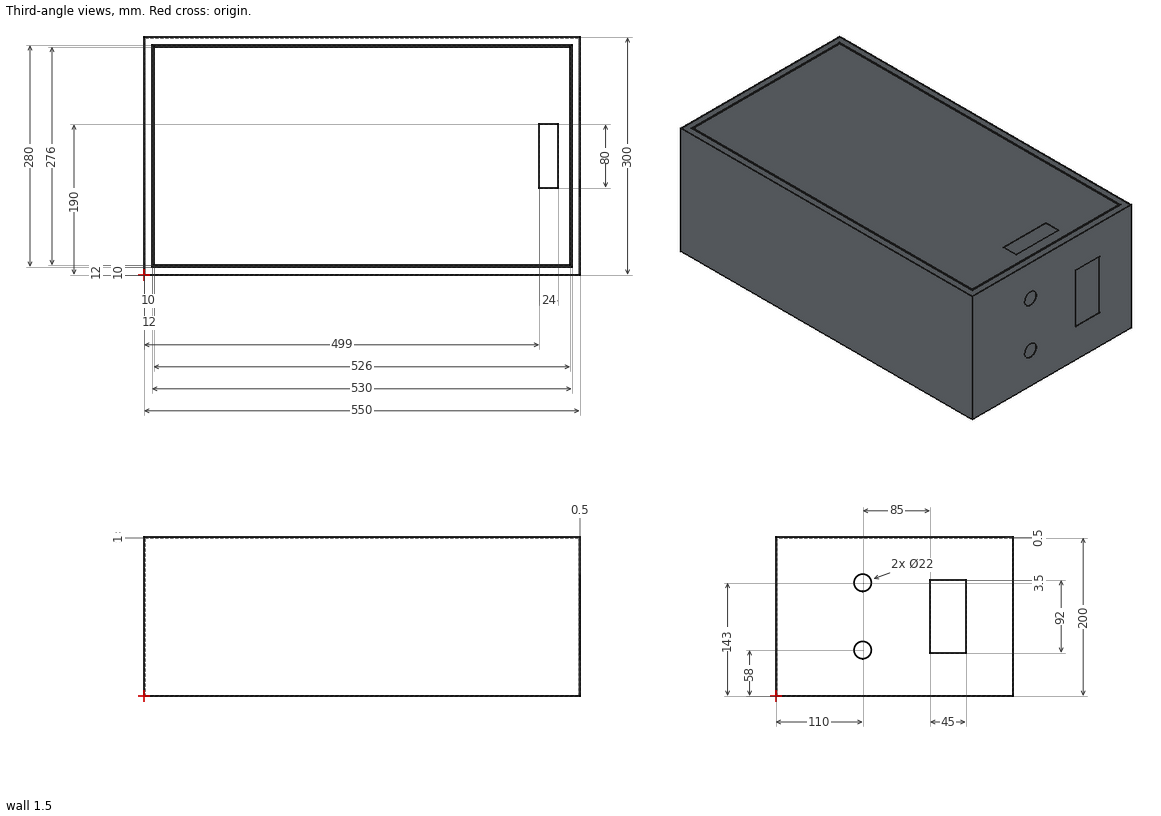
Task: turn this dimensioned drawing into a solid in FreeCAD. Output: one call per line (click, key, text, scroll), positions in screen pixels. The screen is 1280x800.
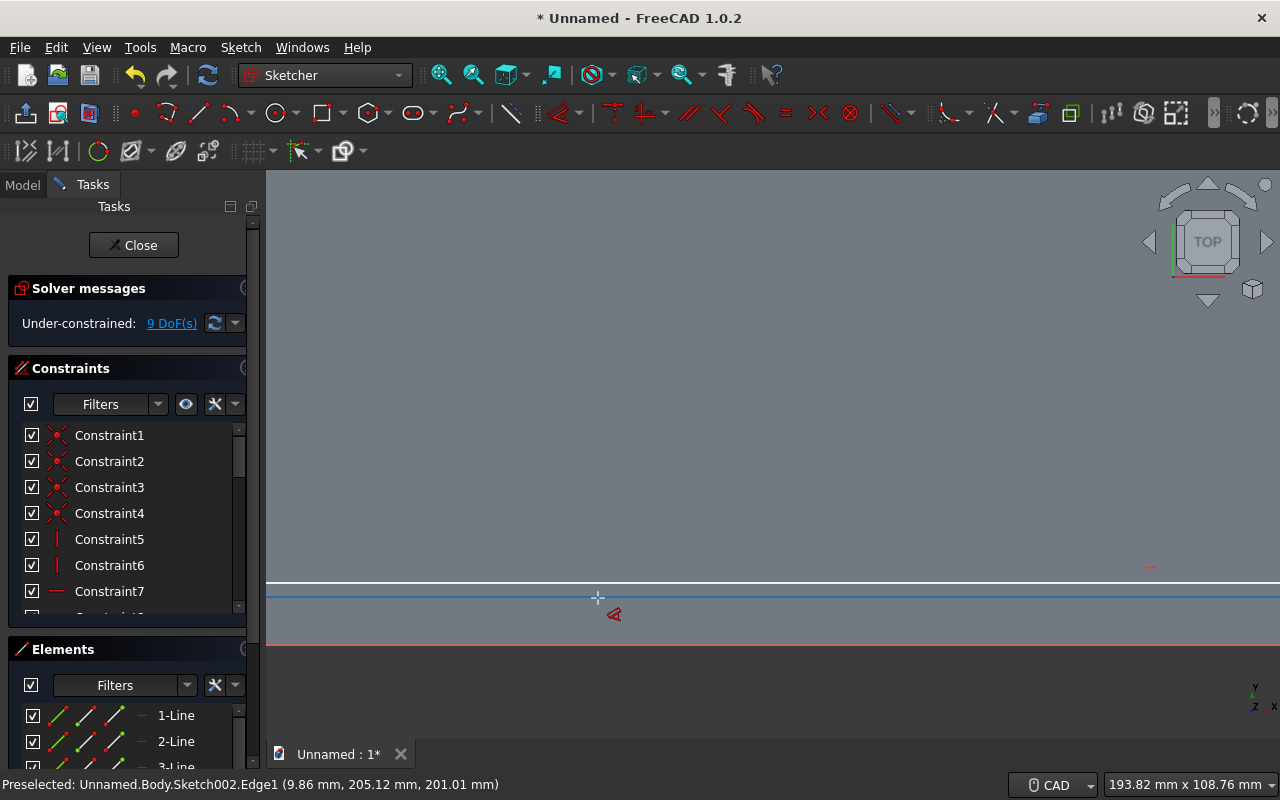
click(598, 597)
click(704, 631)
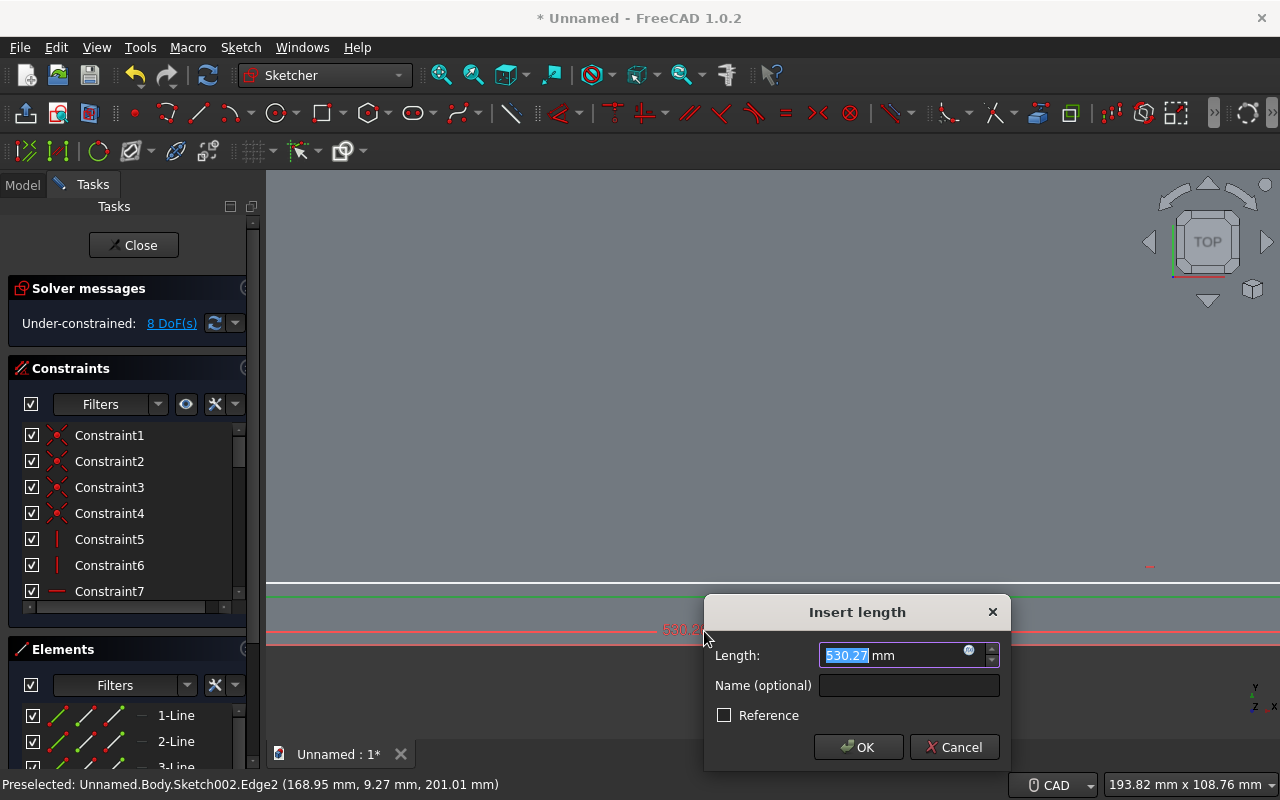
text(530)
key(Return)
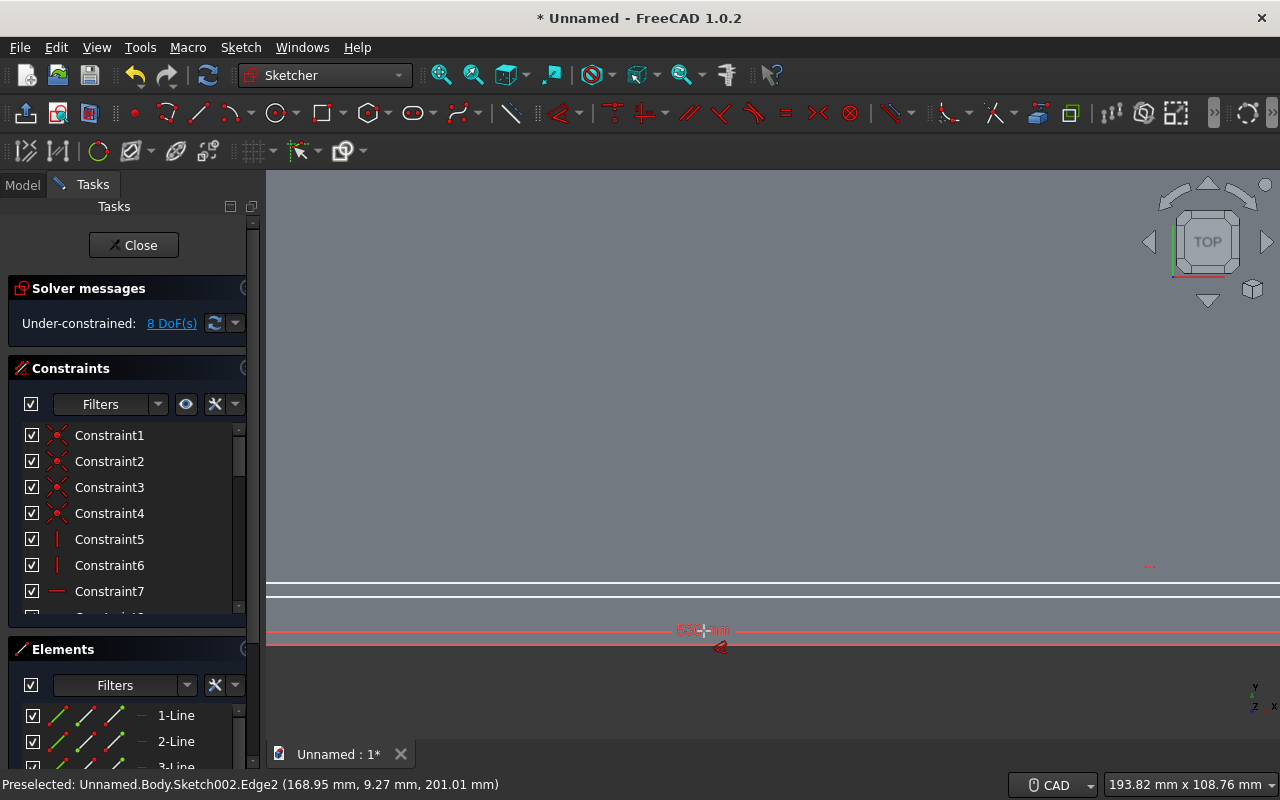
scroll(598, 598, down, 8)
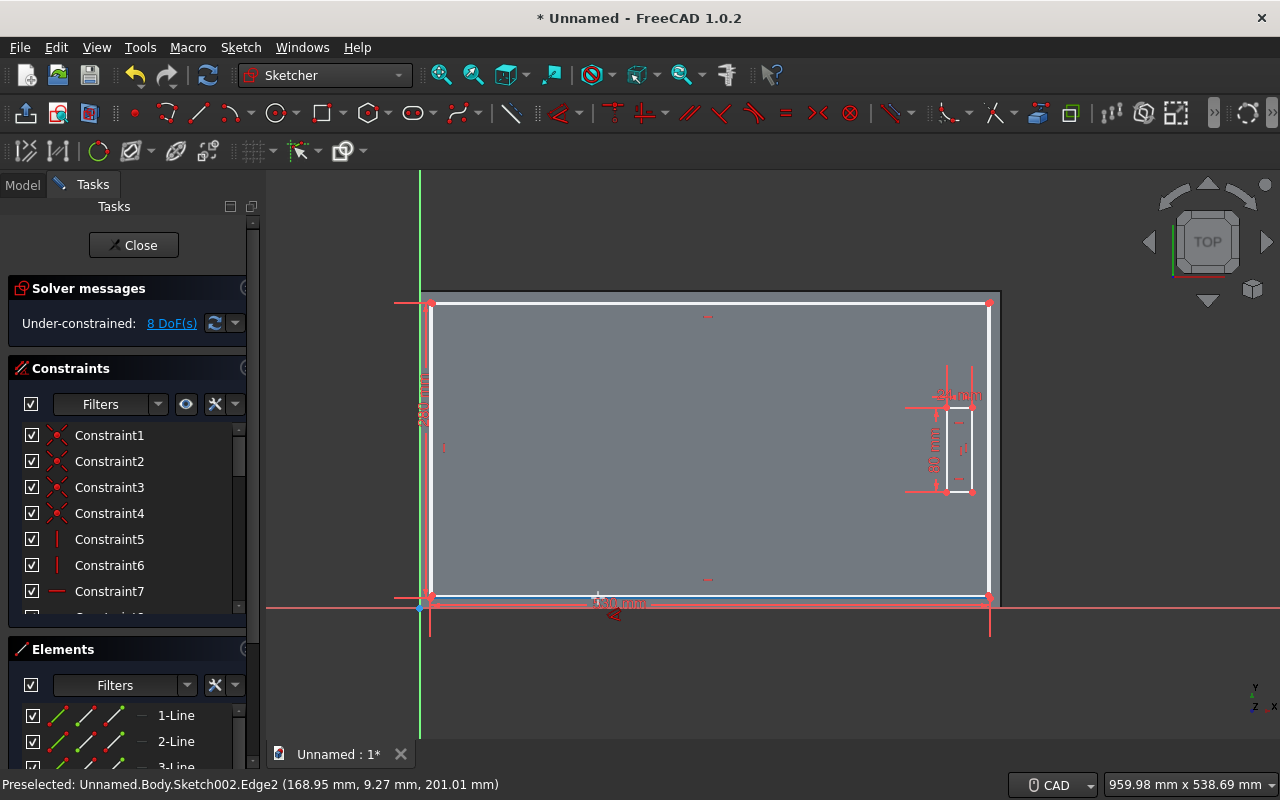
scroll(432, 391, up, 10)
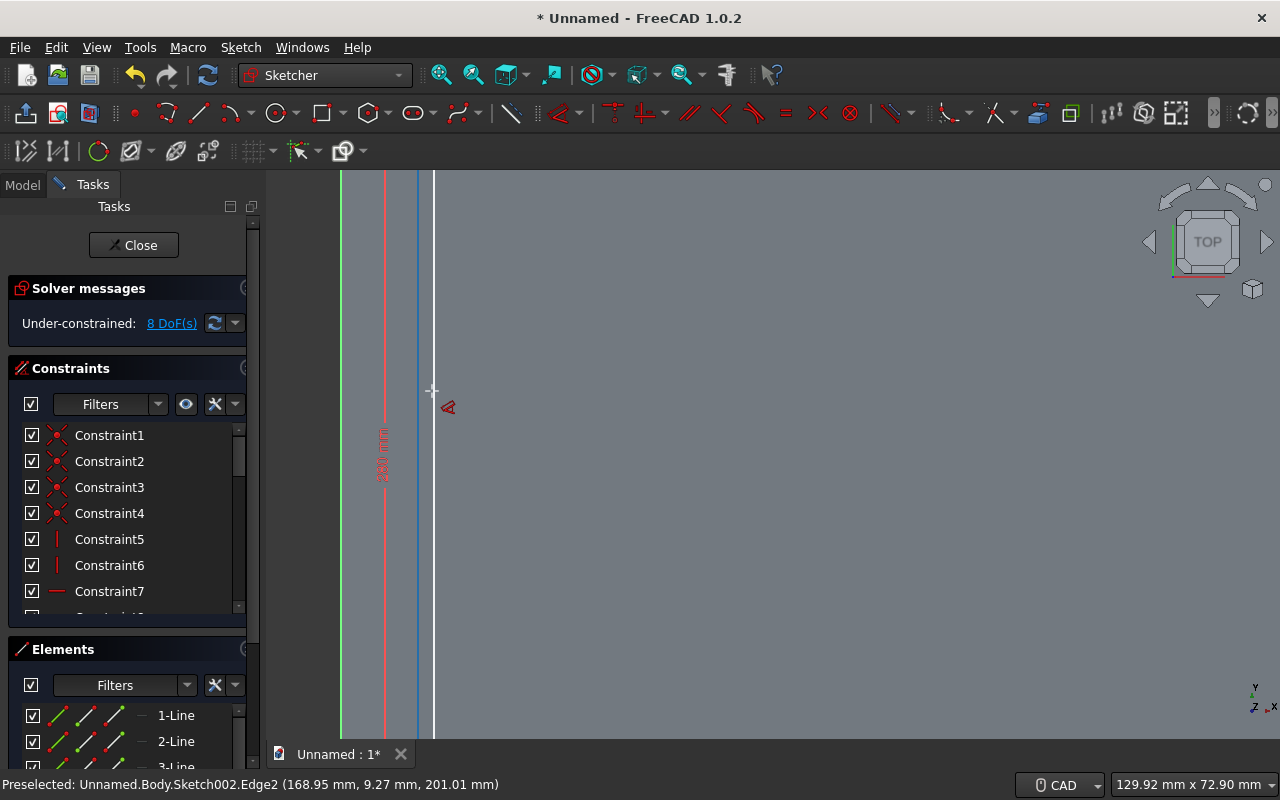
click(434, 392)
click(400, 337)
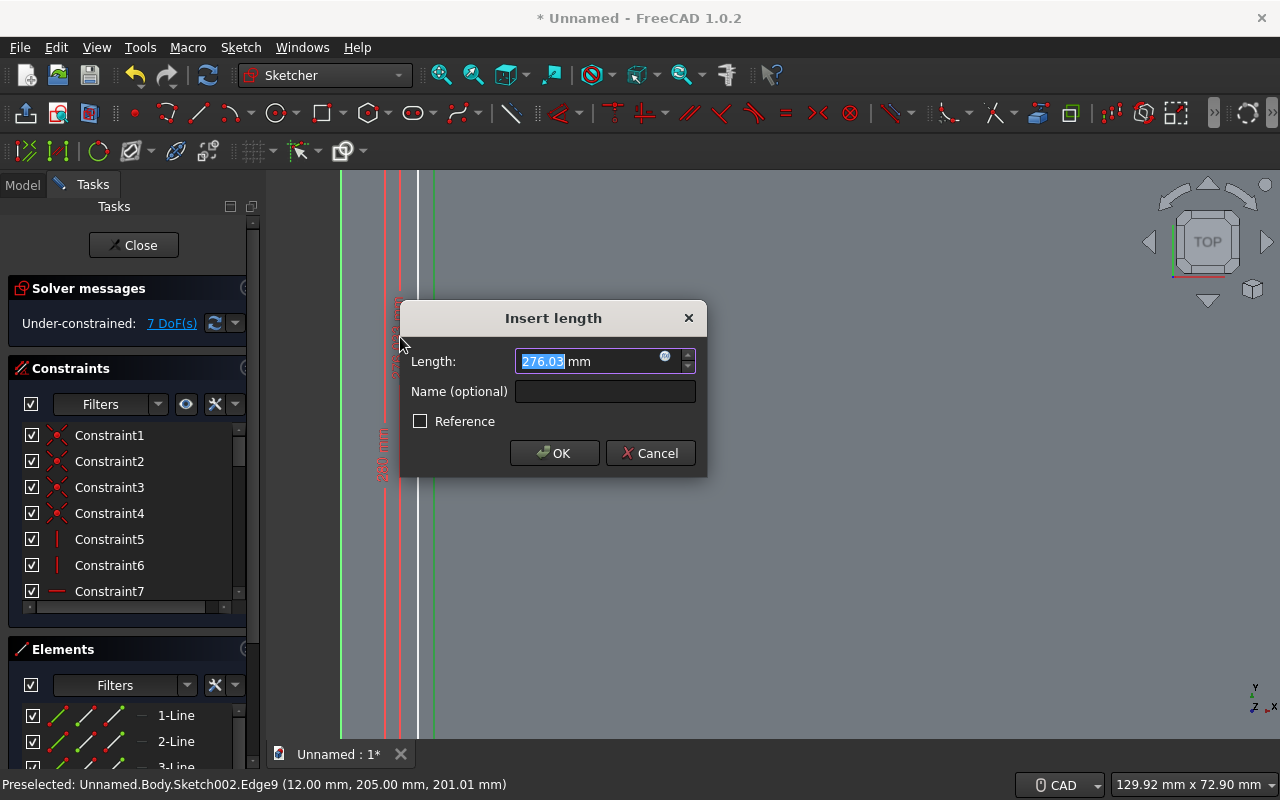
text(276)
key(Return)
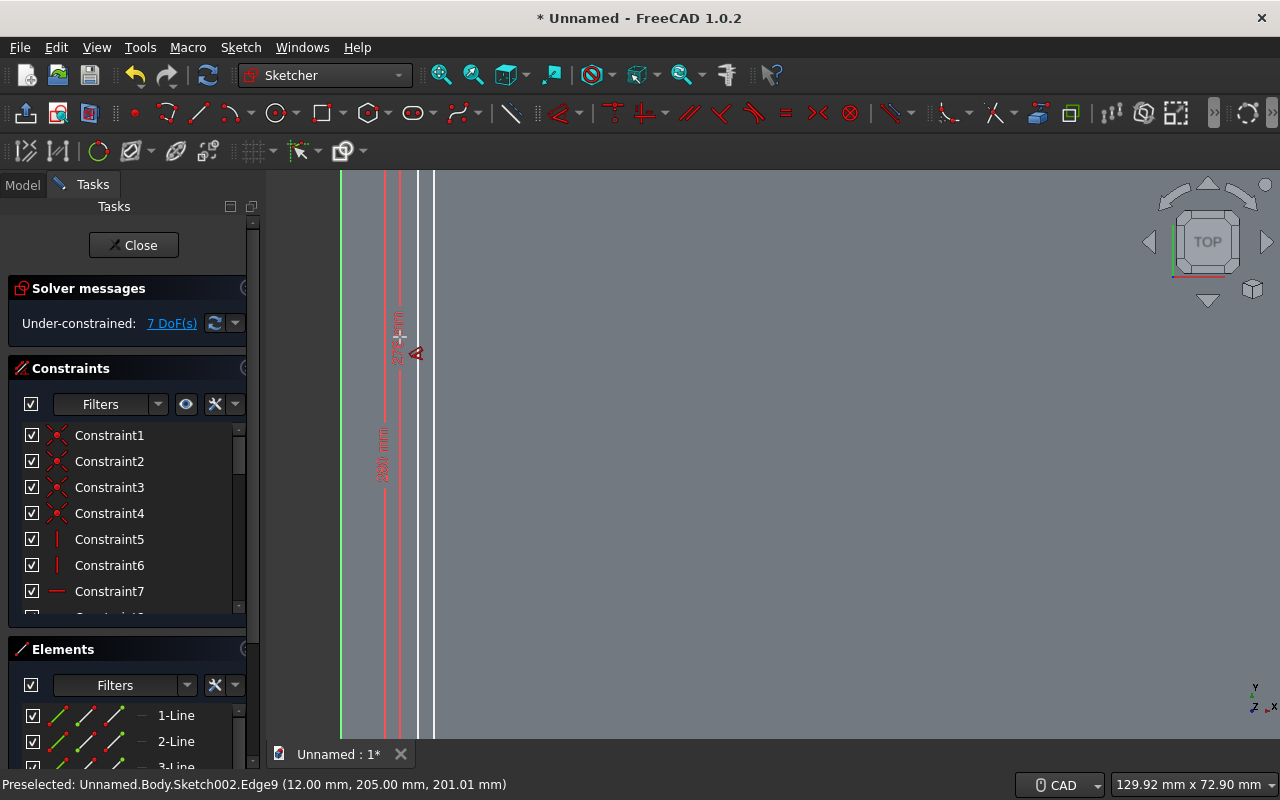
scroll(432, 391, down, 10)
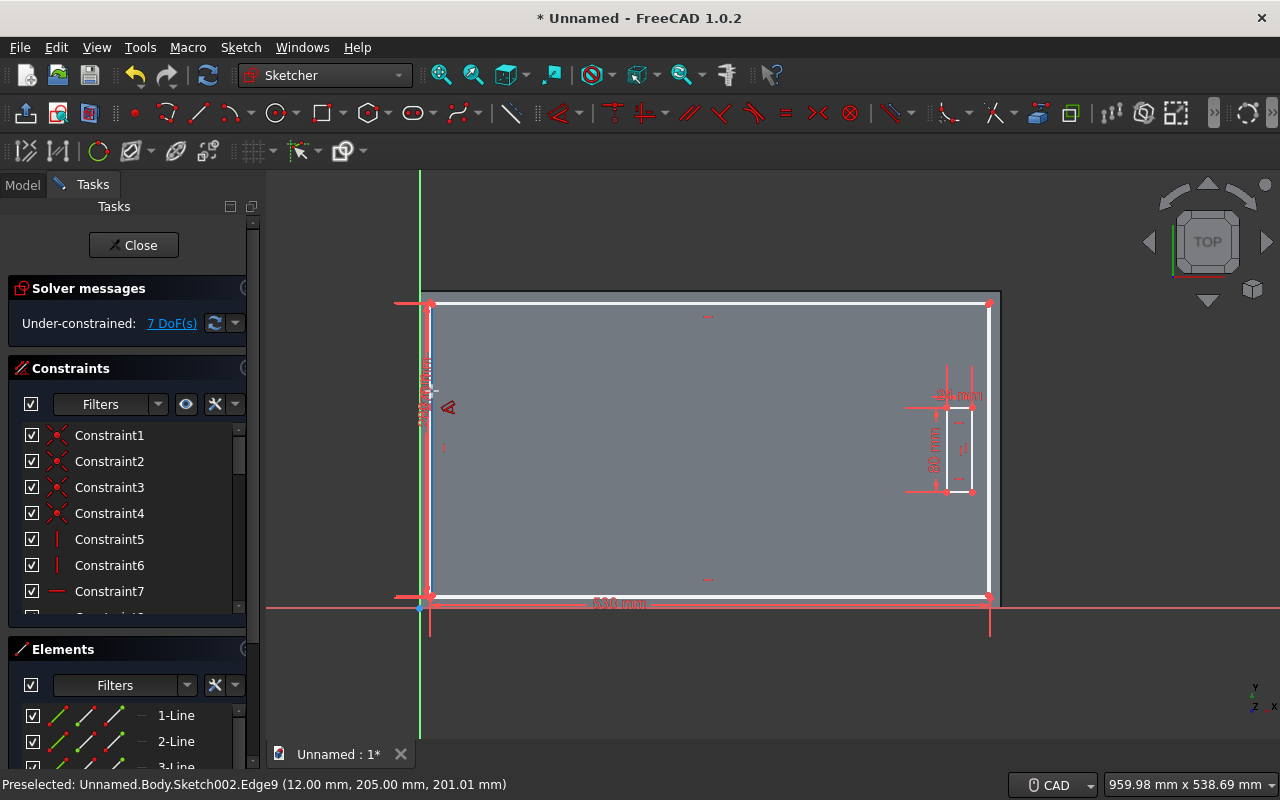
scroll(599, 596, up, 8)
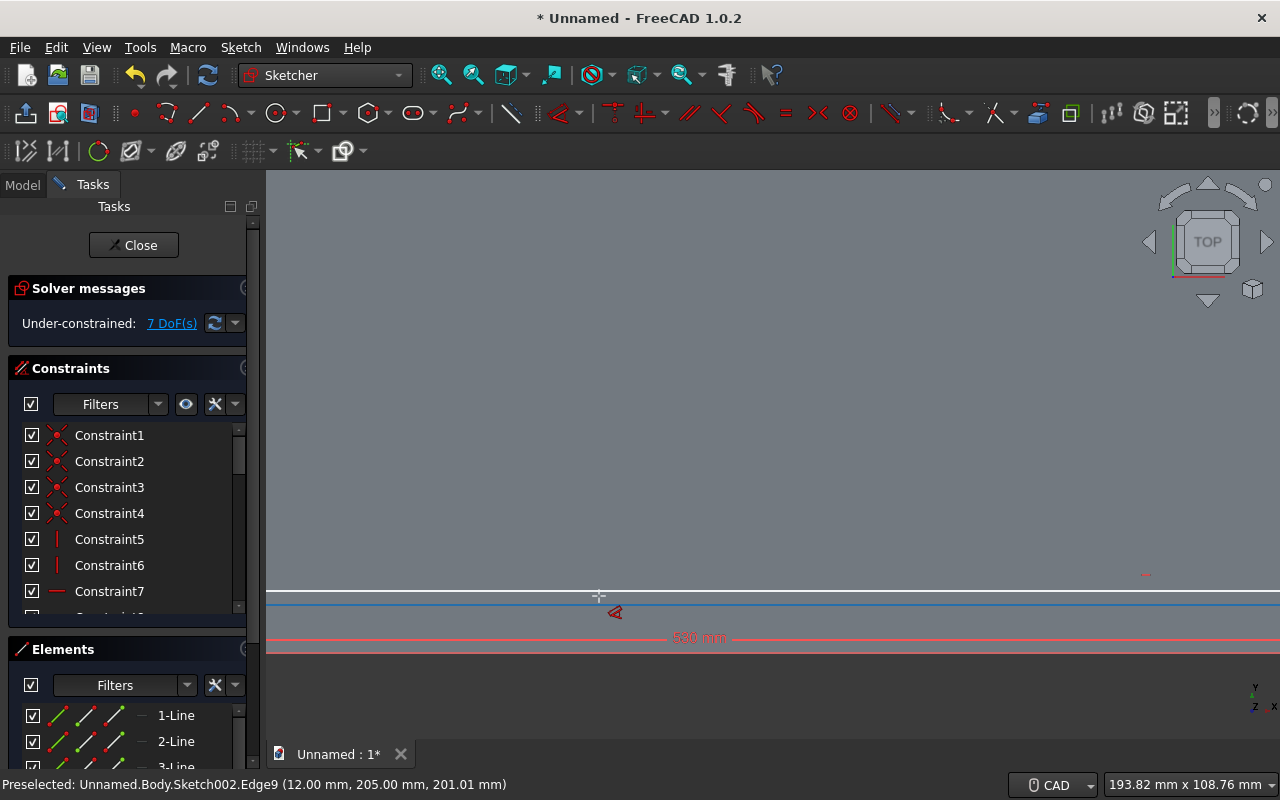
click(598, 591)
click(516, 625)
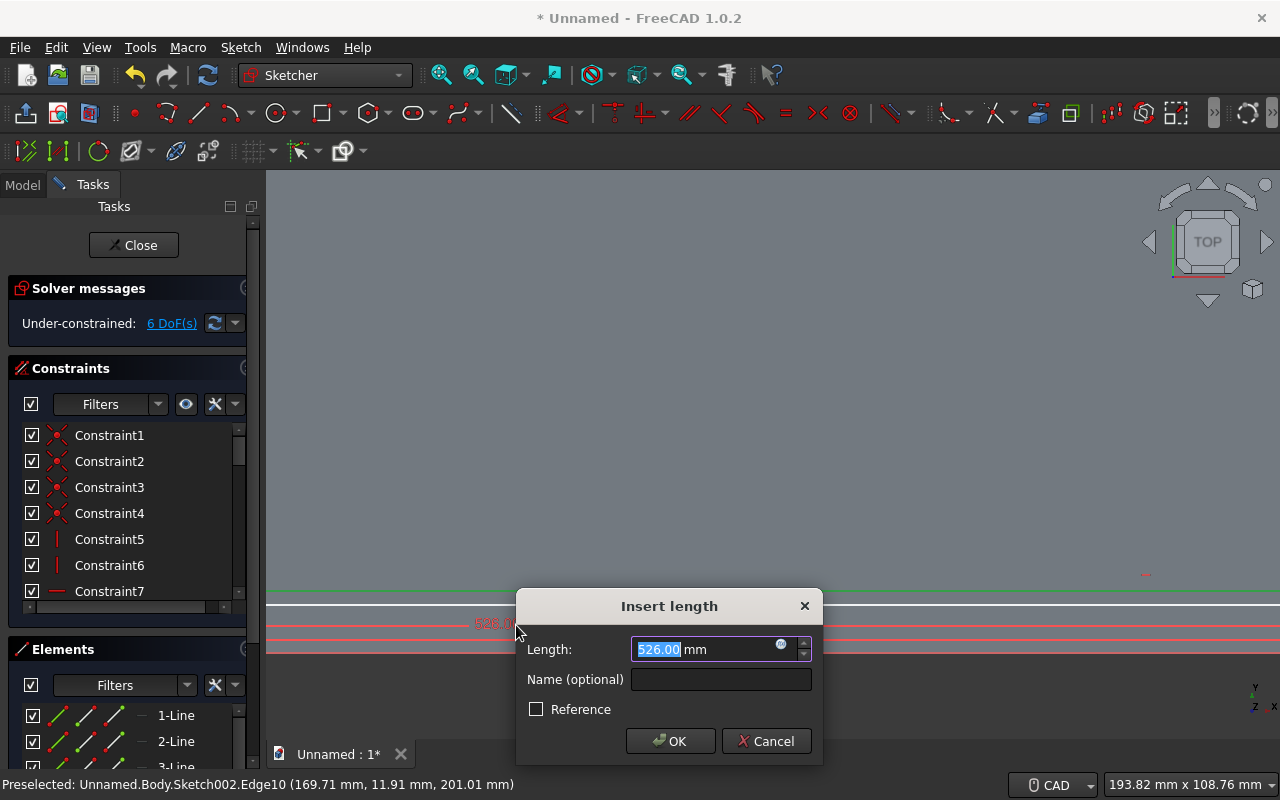
text(526)
key(Return)